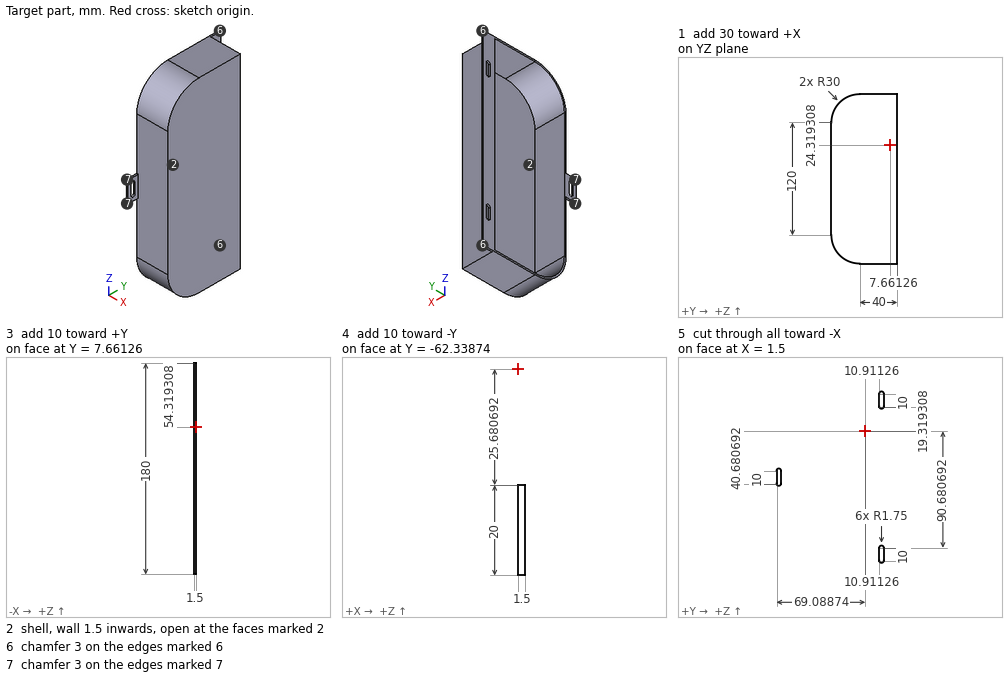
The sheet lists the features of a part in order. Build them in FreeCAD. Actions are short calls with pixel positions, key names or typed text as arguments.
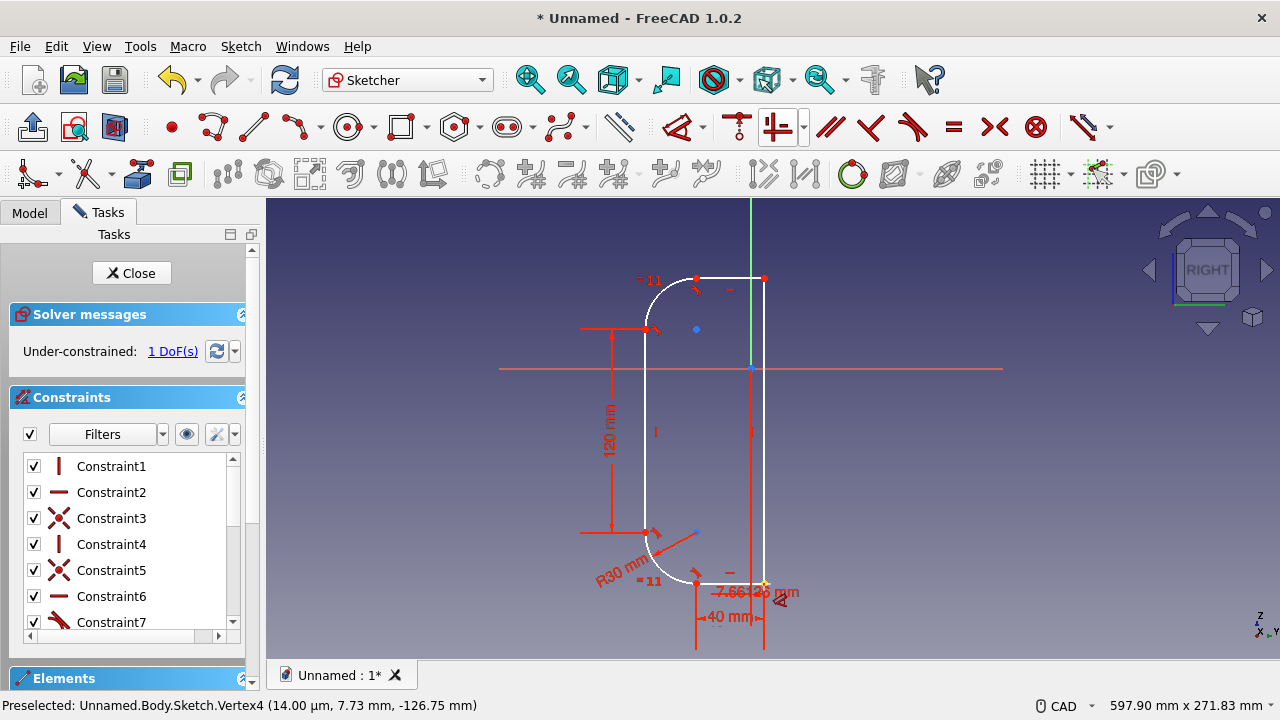
click(645, 329)
click(611, 349)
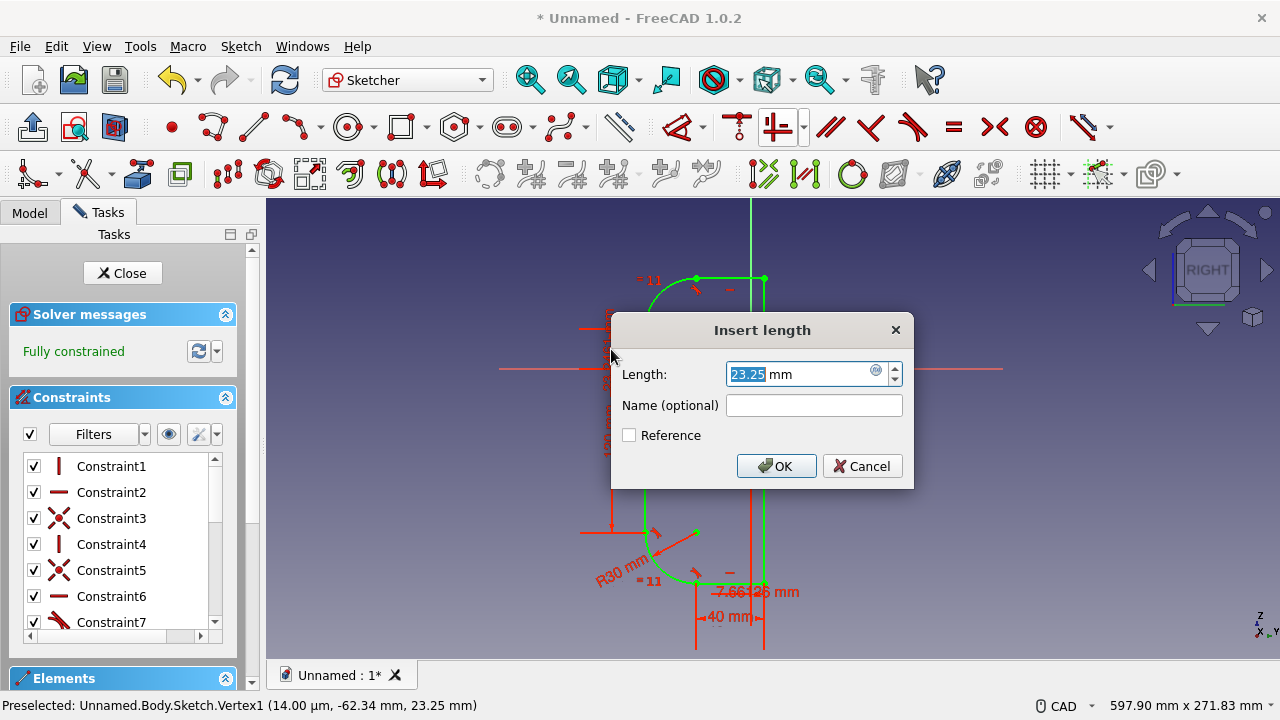
text(24.319308)
key(Return)
key(Escape)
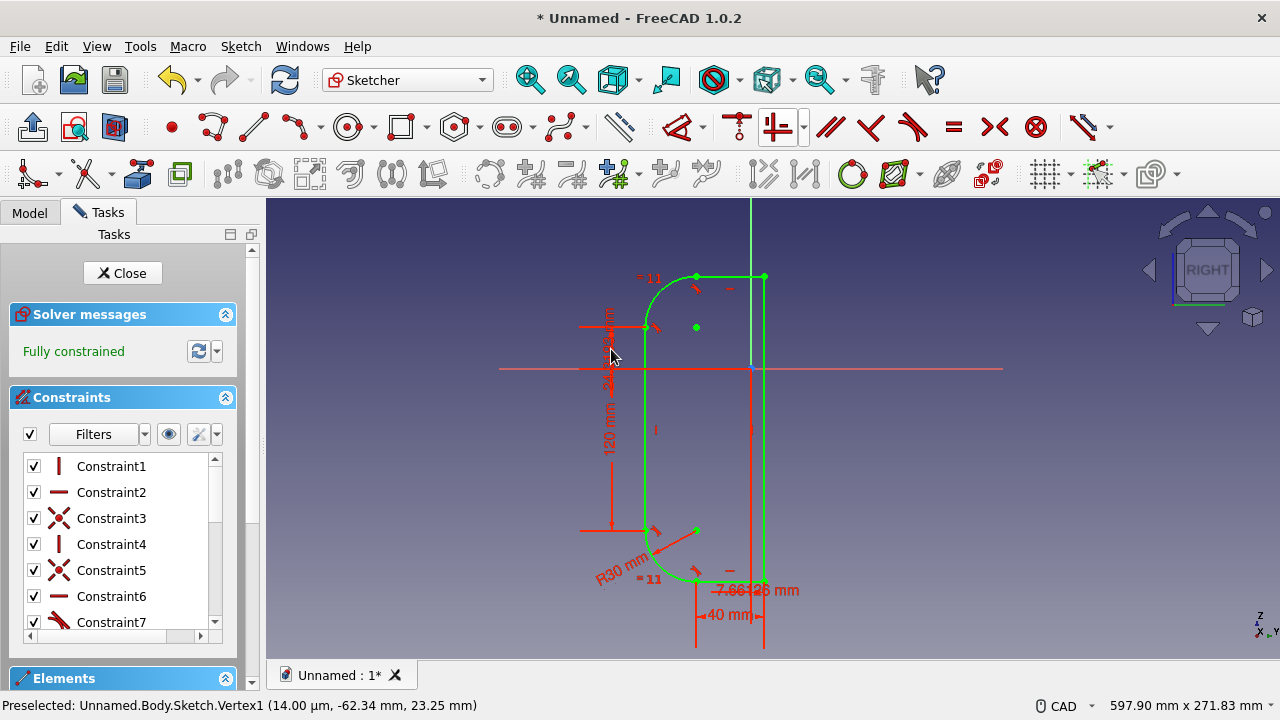
click(123, 273)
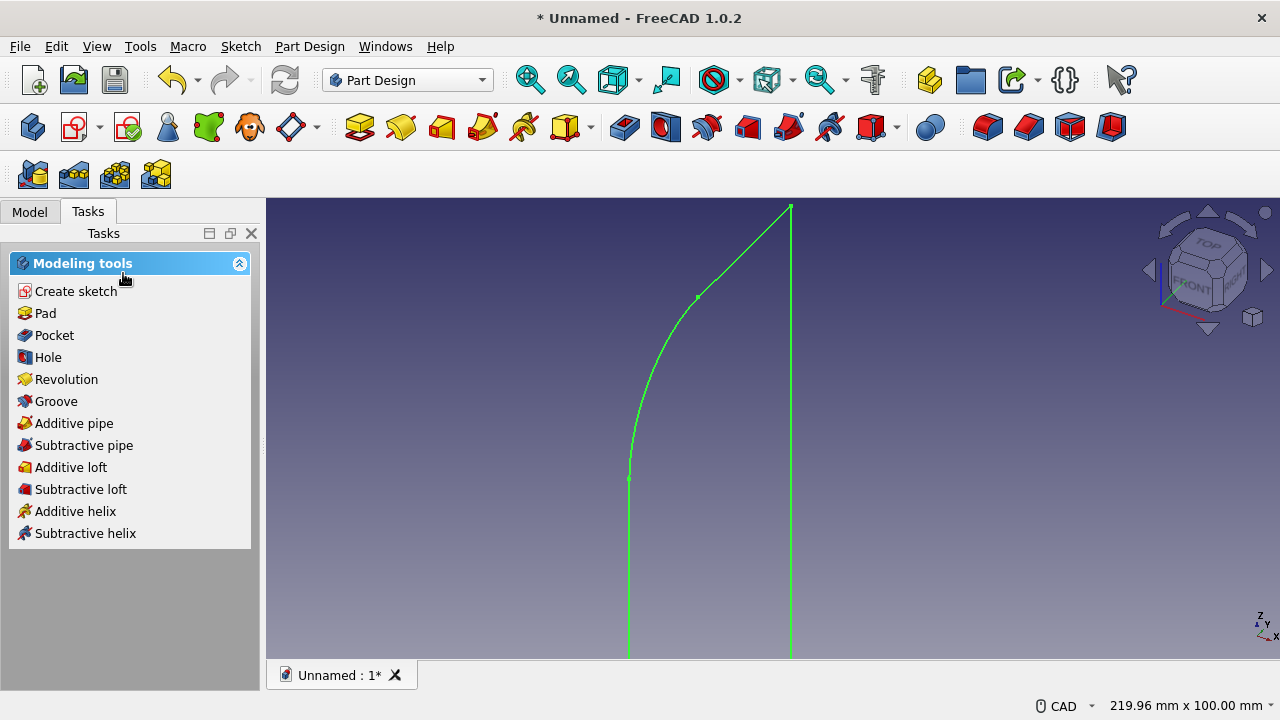
click(360, 128)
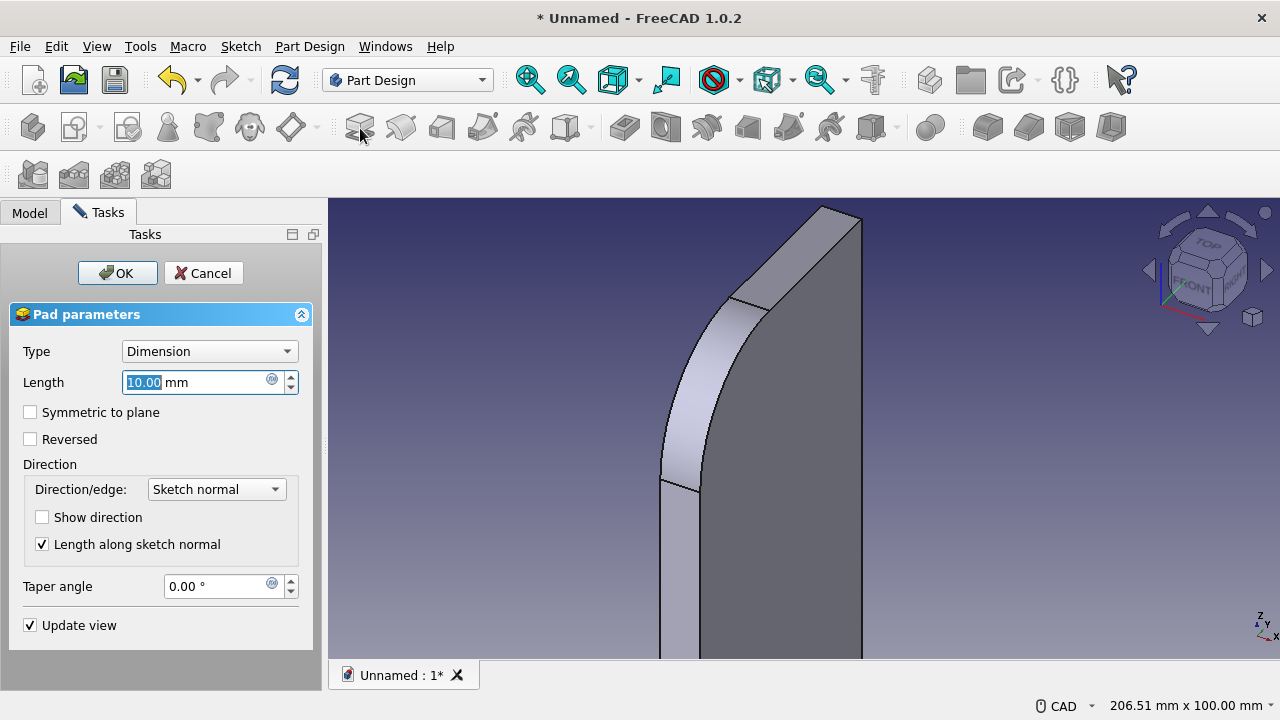
text(30)
key(Tab)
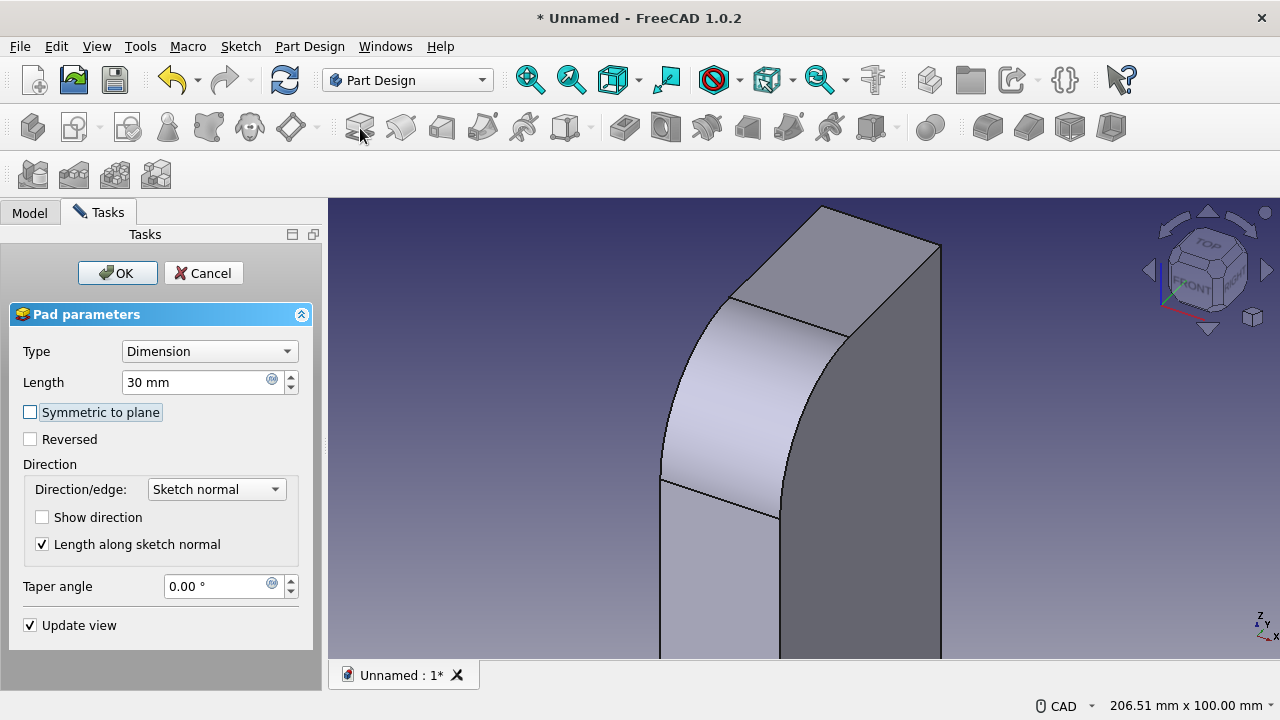
click(118, 273)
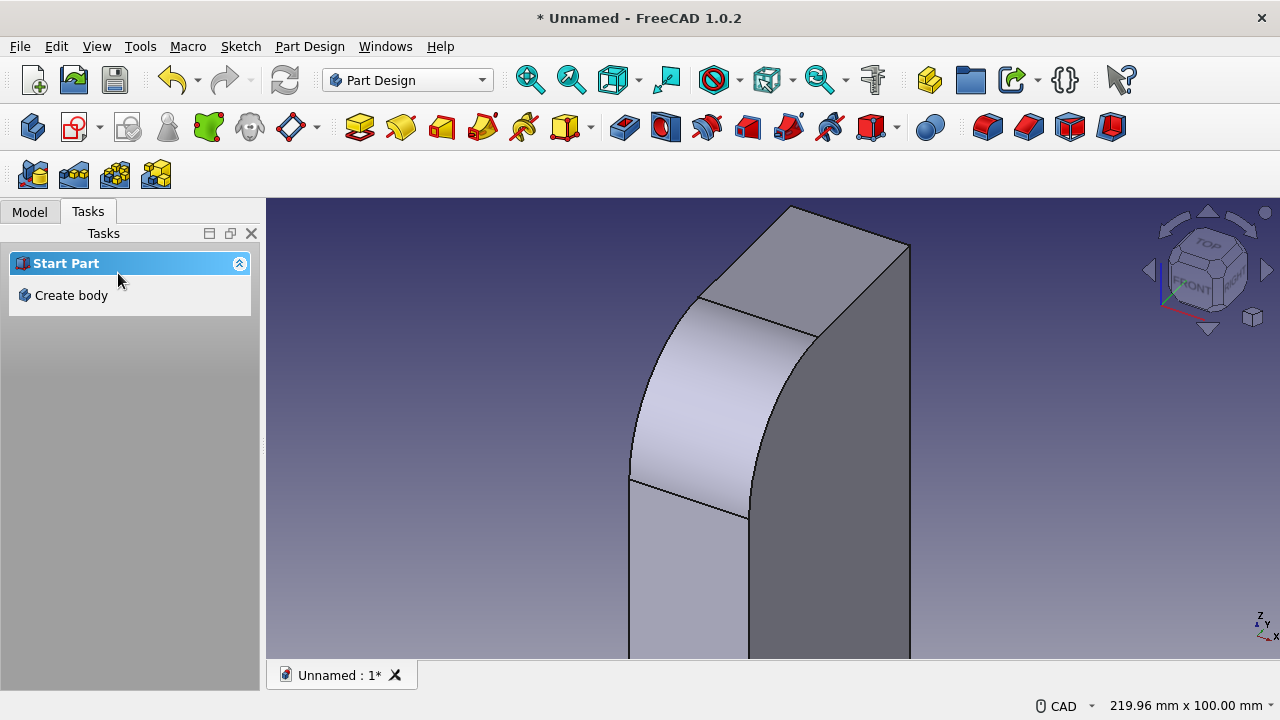
click(531, 80)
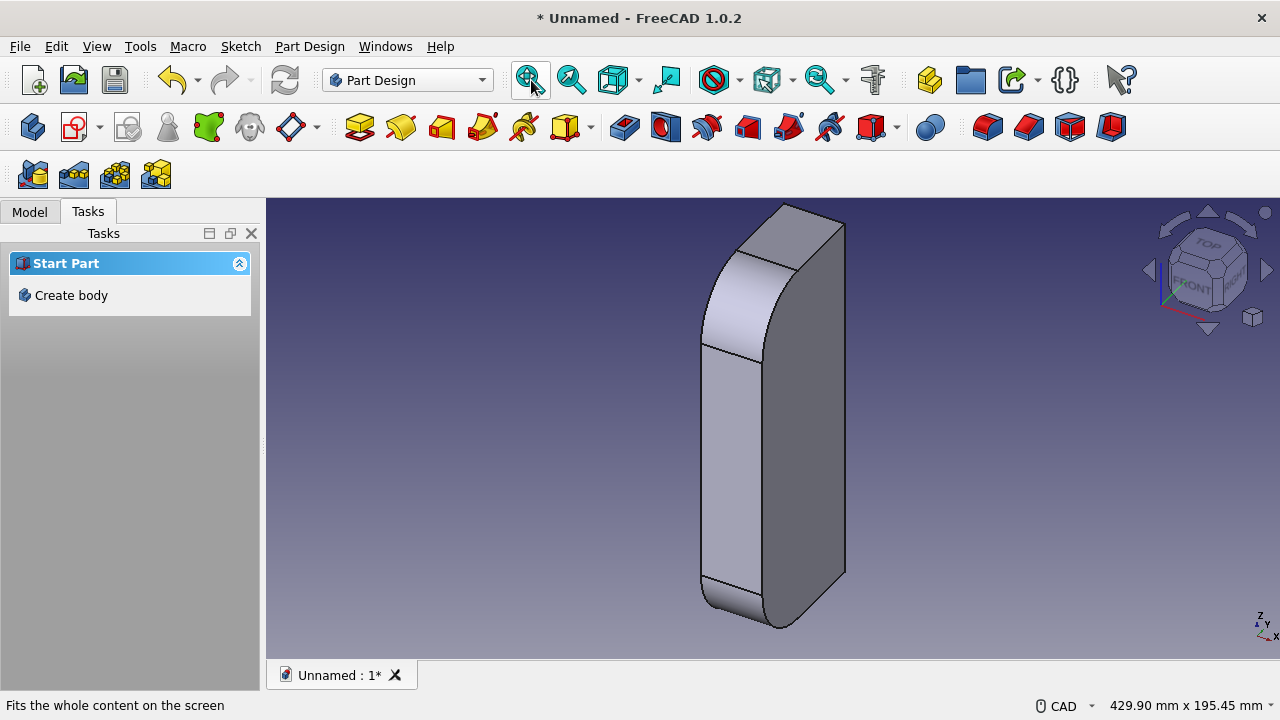
key(0)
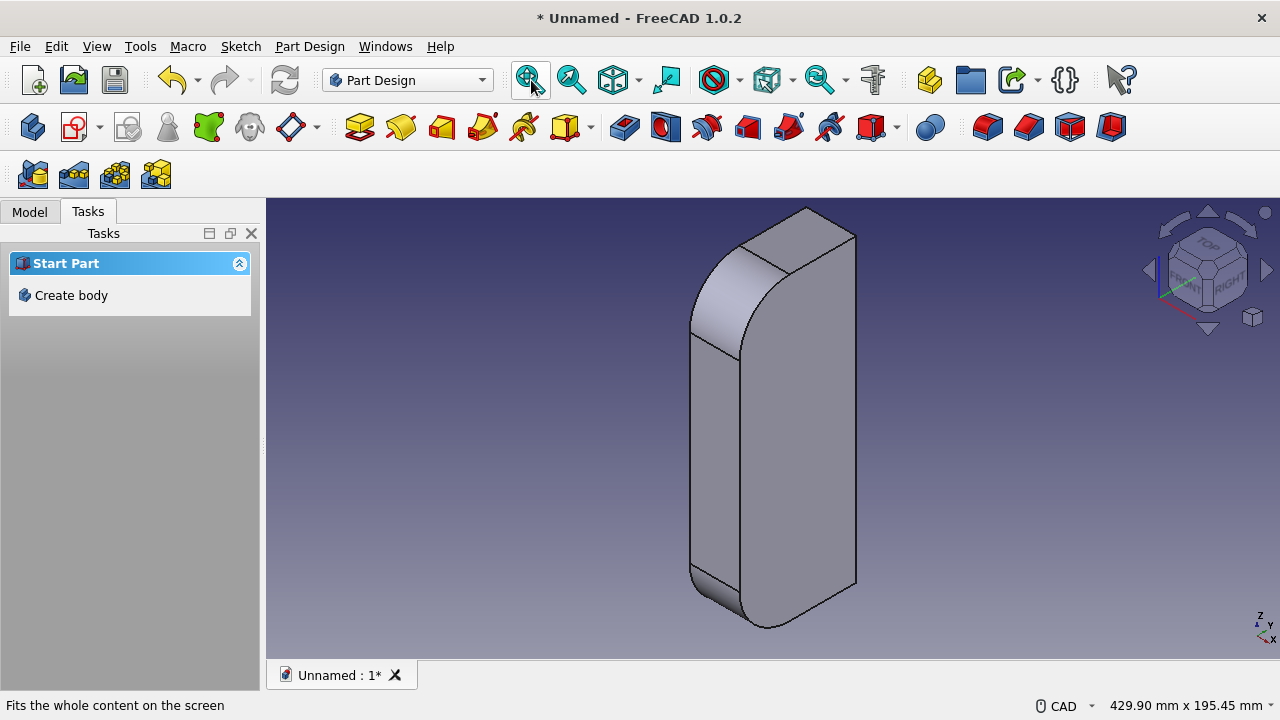
key(2)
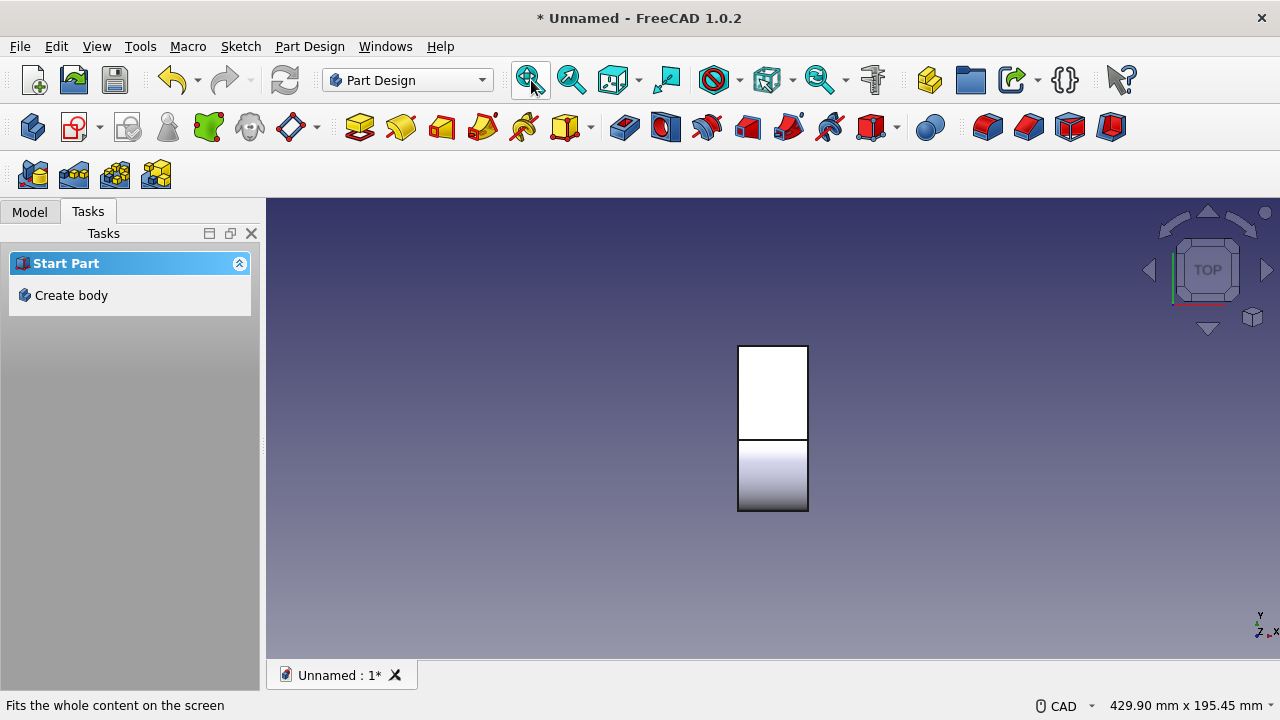
click(531, 80)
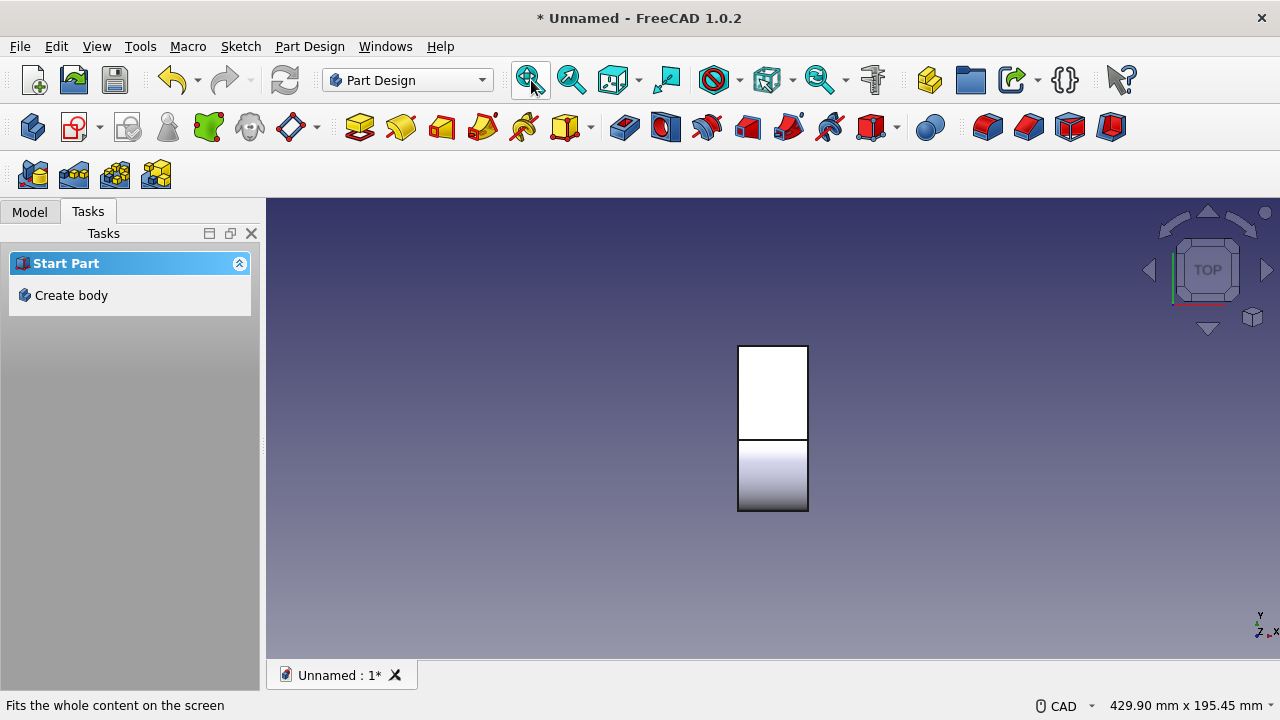
key(1)